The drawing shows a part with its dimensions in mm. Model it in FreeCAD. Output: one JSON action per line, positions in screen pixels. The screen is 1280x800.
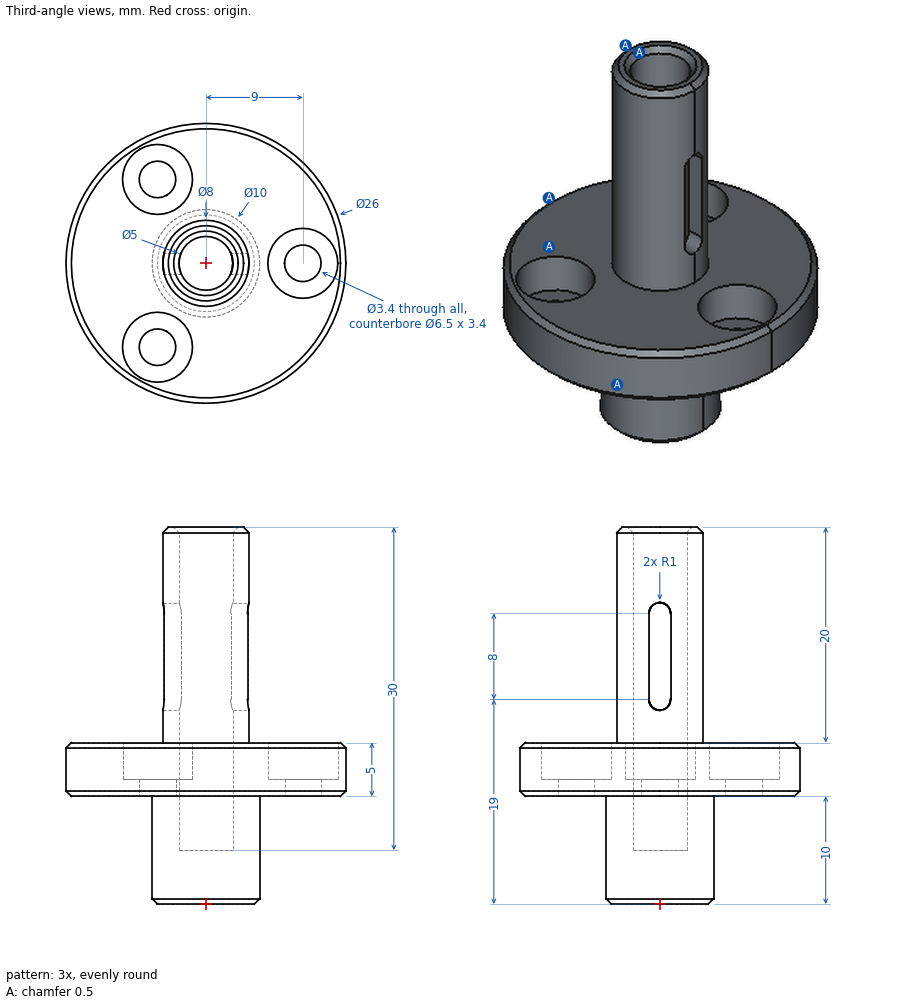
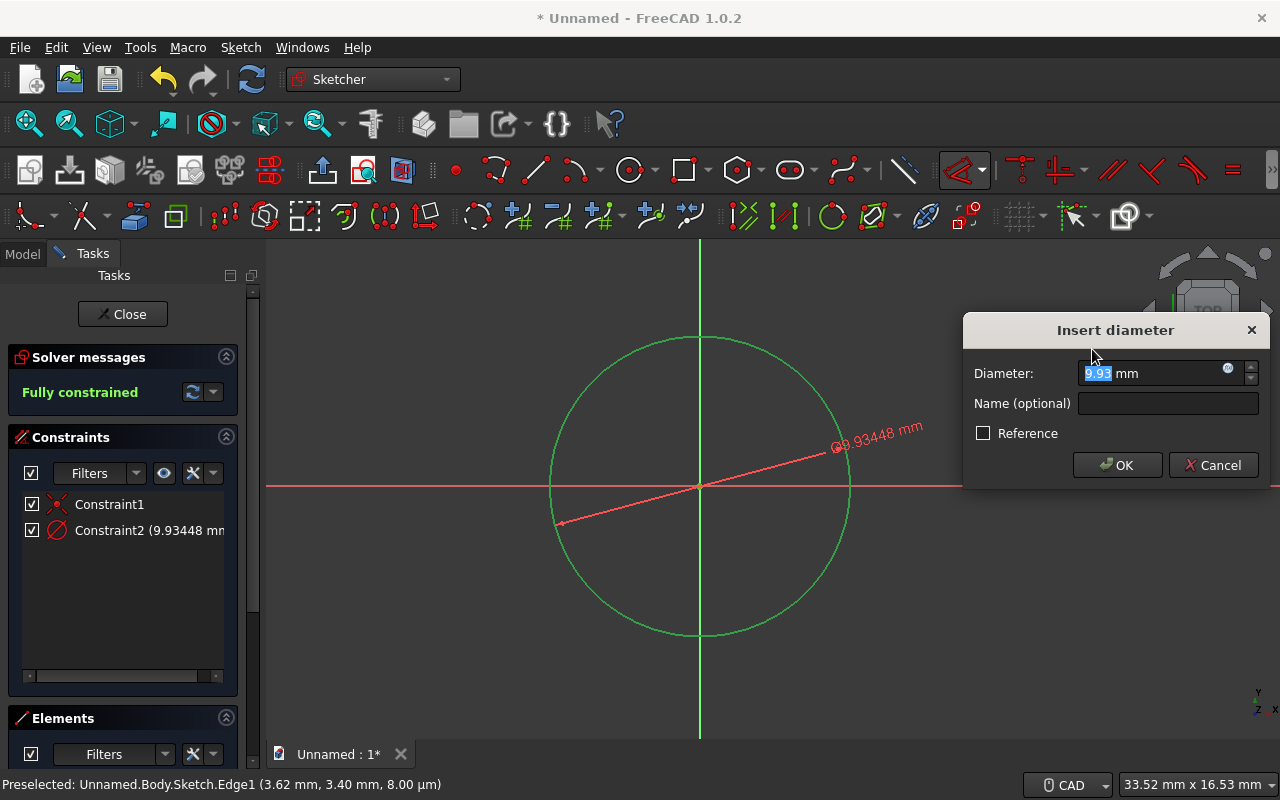
{"action": "type", "text": "10"}
{"action": "key", "text": "Return"}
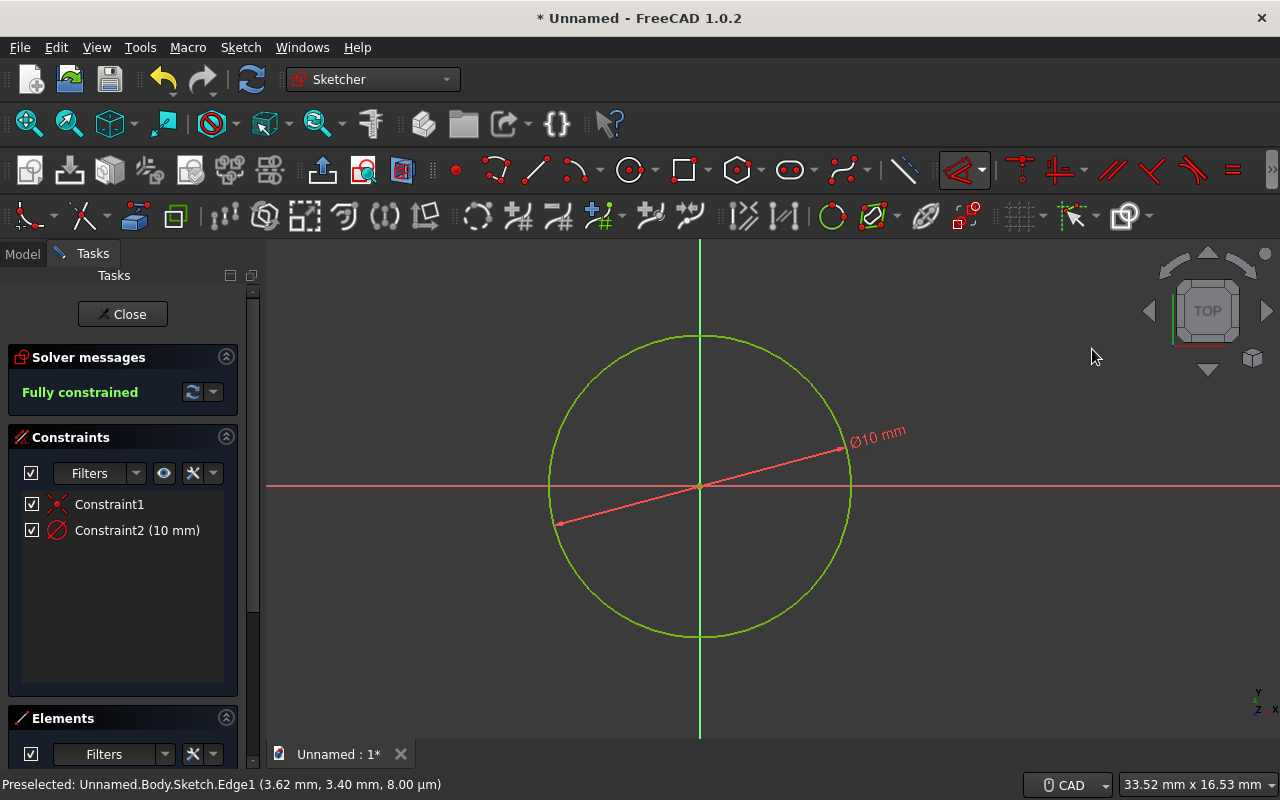
{"action": "left_click", "coordinate": [123, 314]}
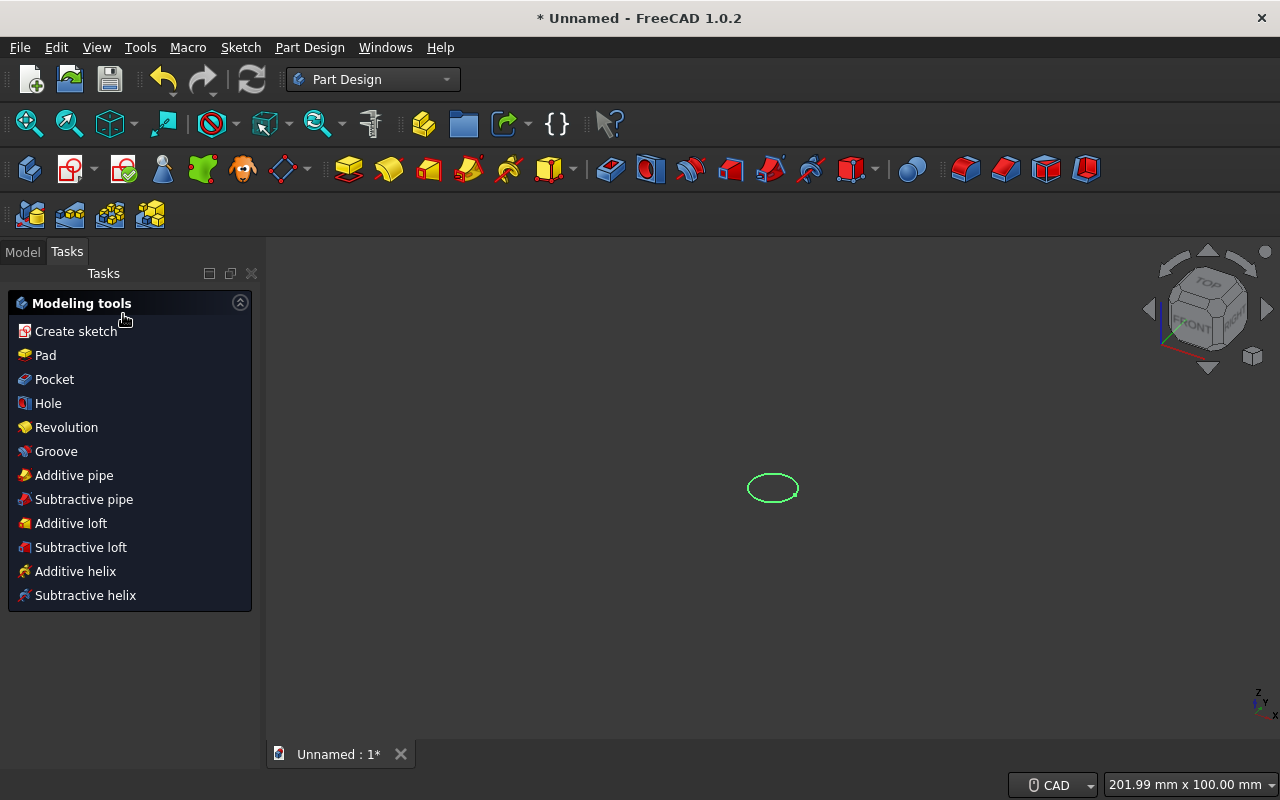
{"action": "left_click", "coordinate": [350, 170]}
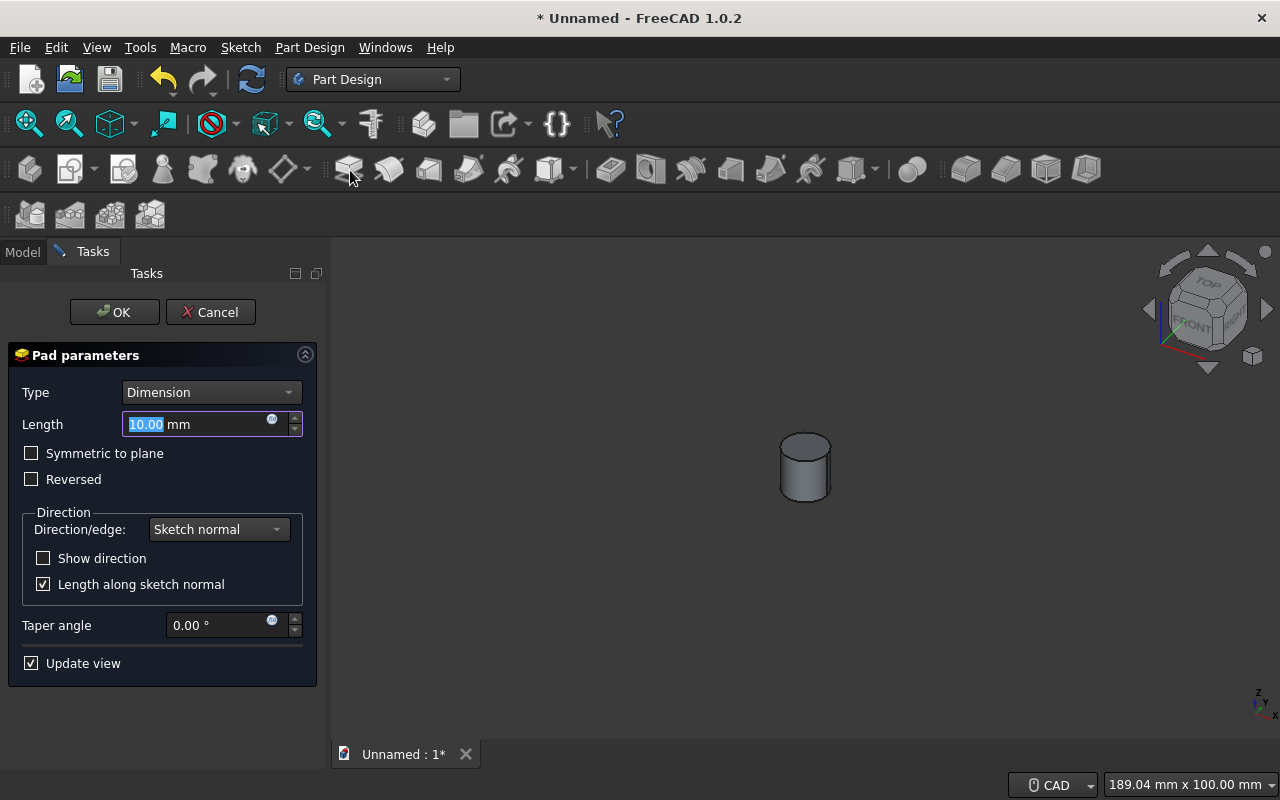
{"action": "type", "text": "10"}
{"action": "key", "text": "Tab"}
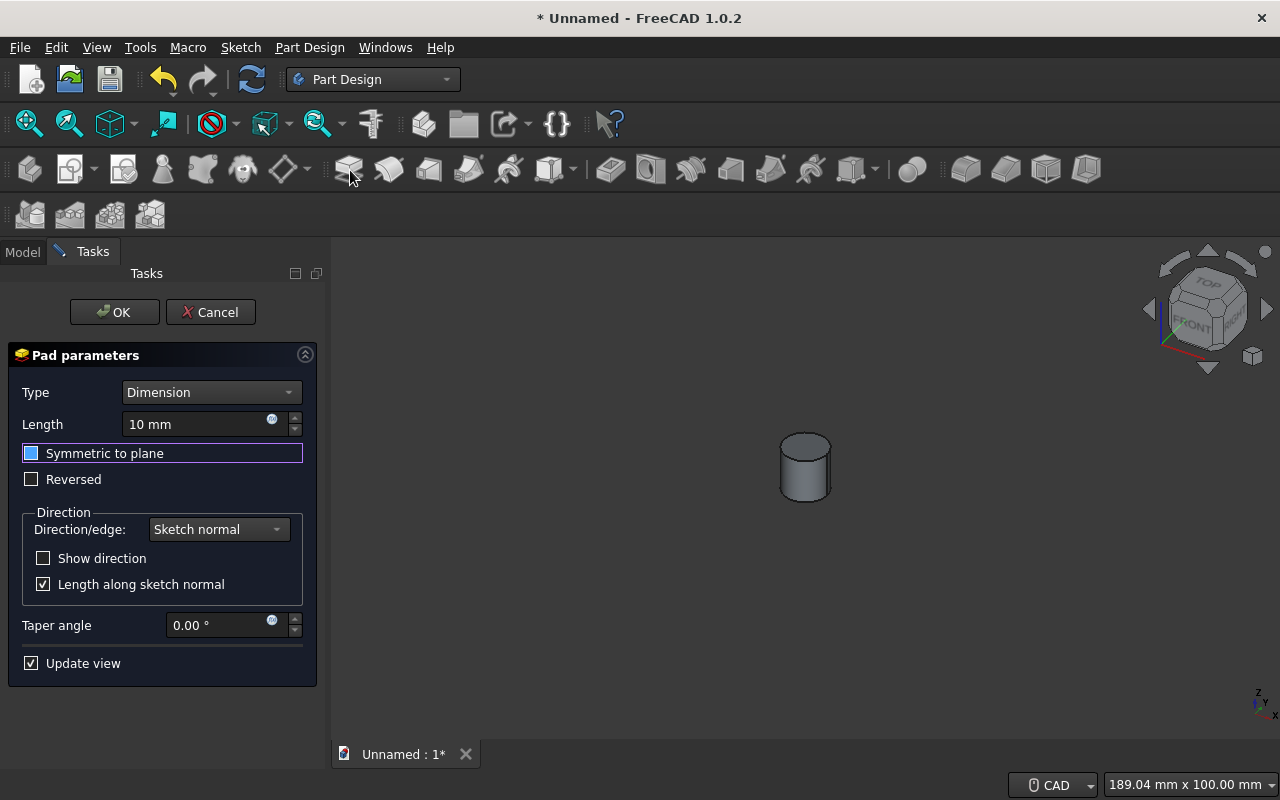
{"action": "left_click", "coordinate": [115, 312]}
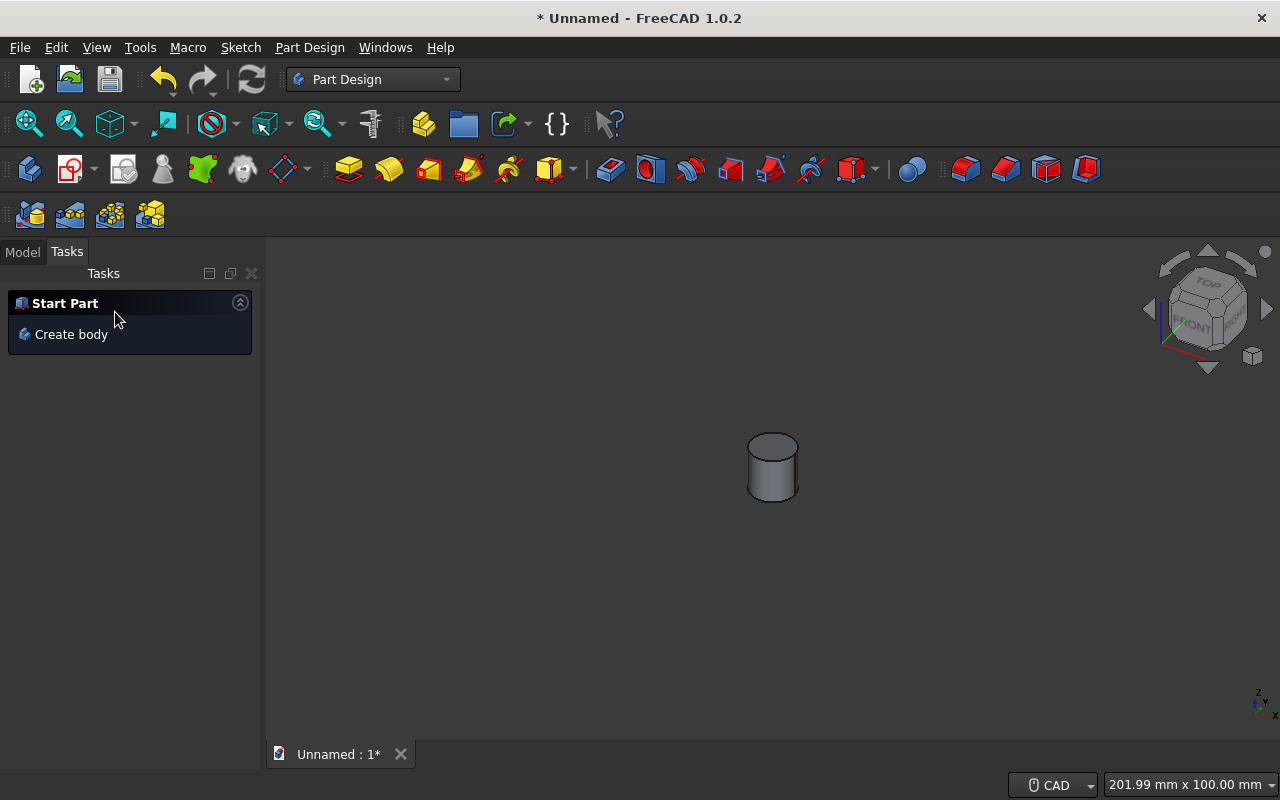
{"action": "left_click", "coordinate": [30, 124]}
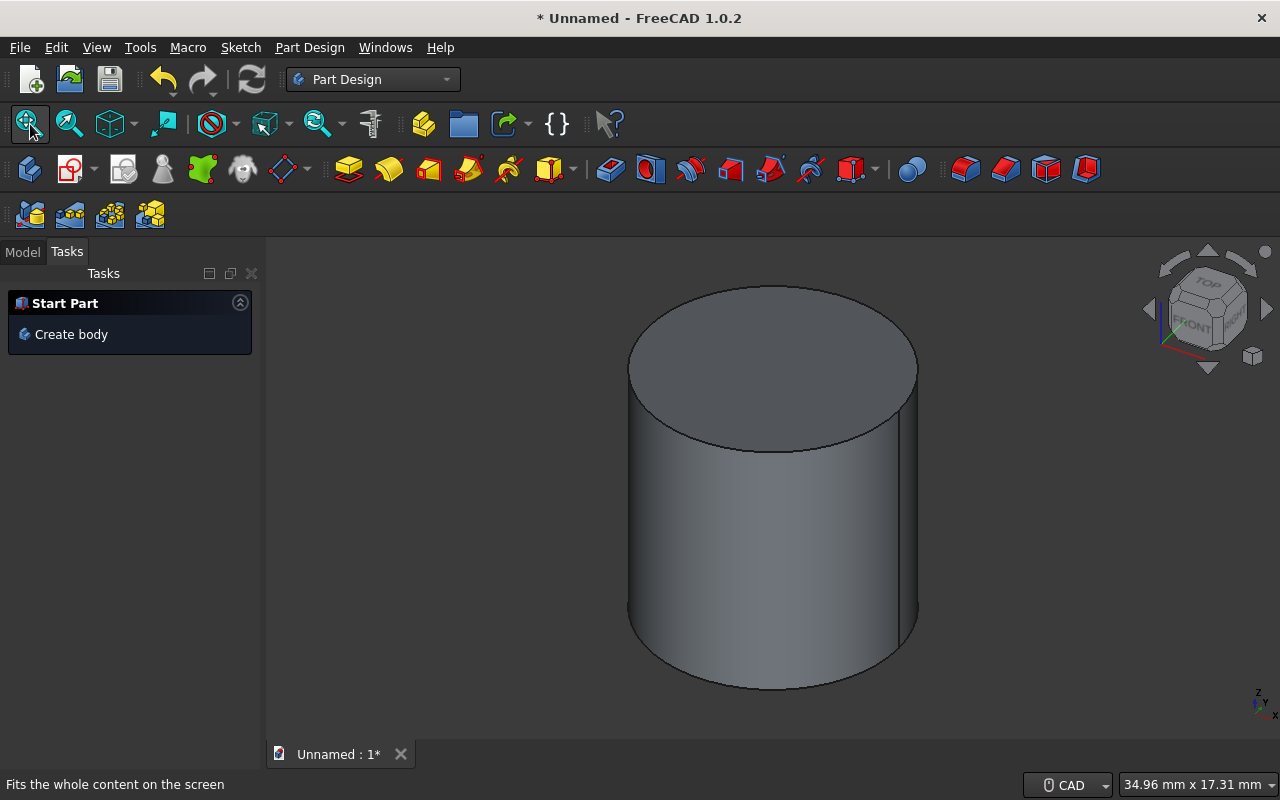
{"action": "left_click", "coordinate": [773, 368]}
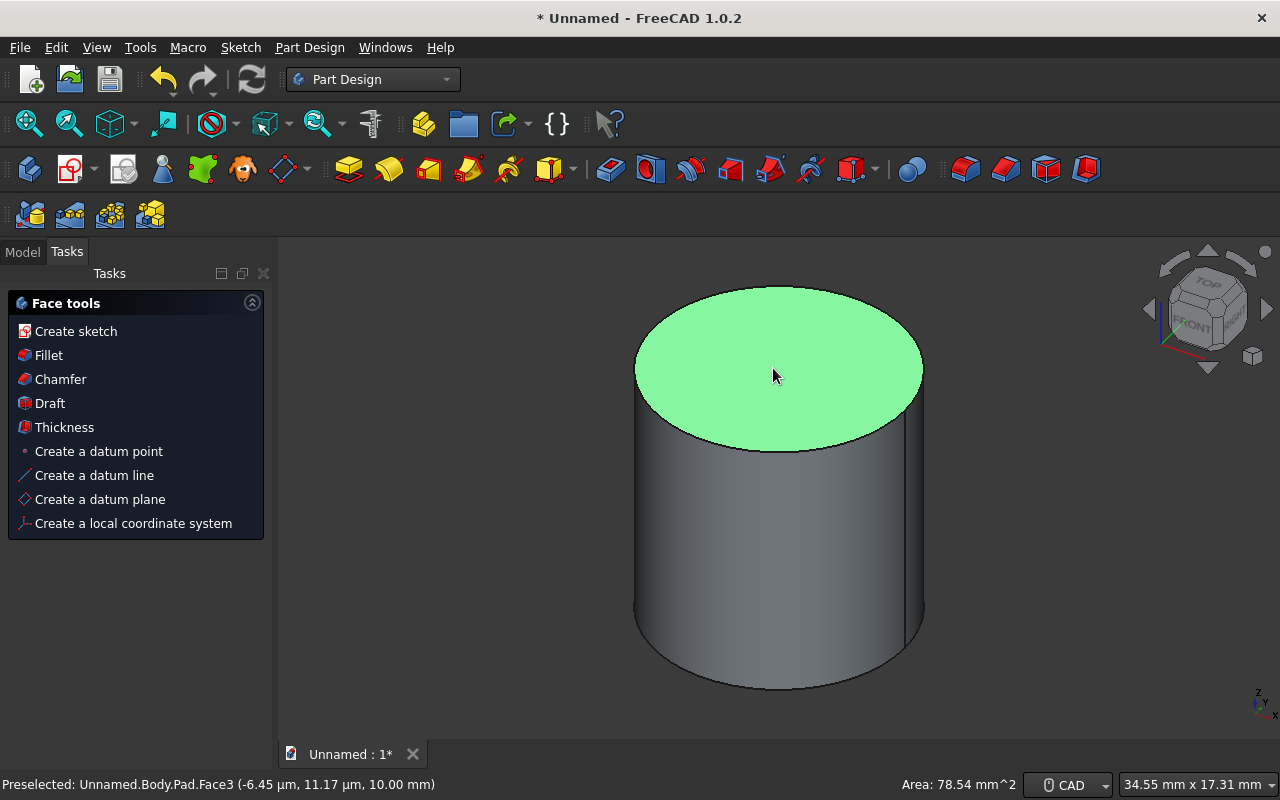
{"action": "left_click", "coordinate": [70, 170]}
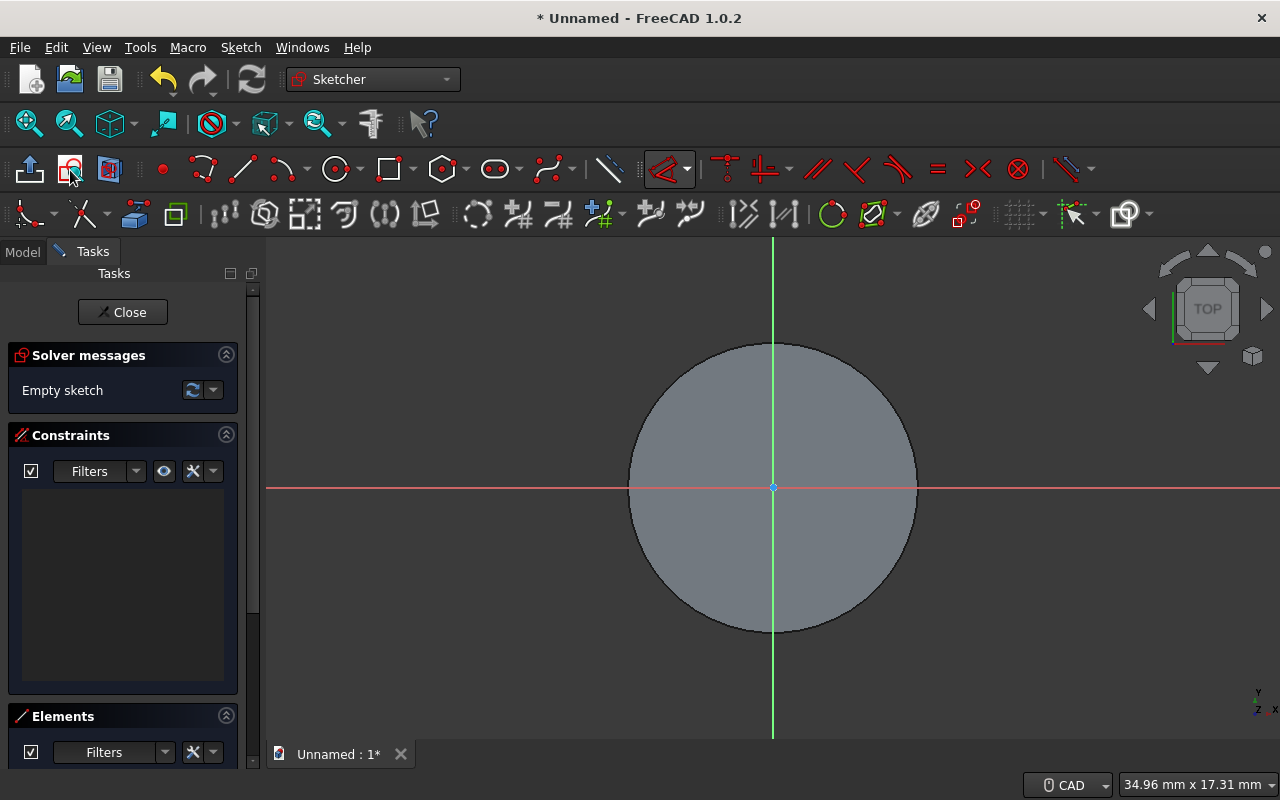
{"action": "scroll", "coordinate": [649, 488], "scroll_direction": "down", "scroll_amount": 4}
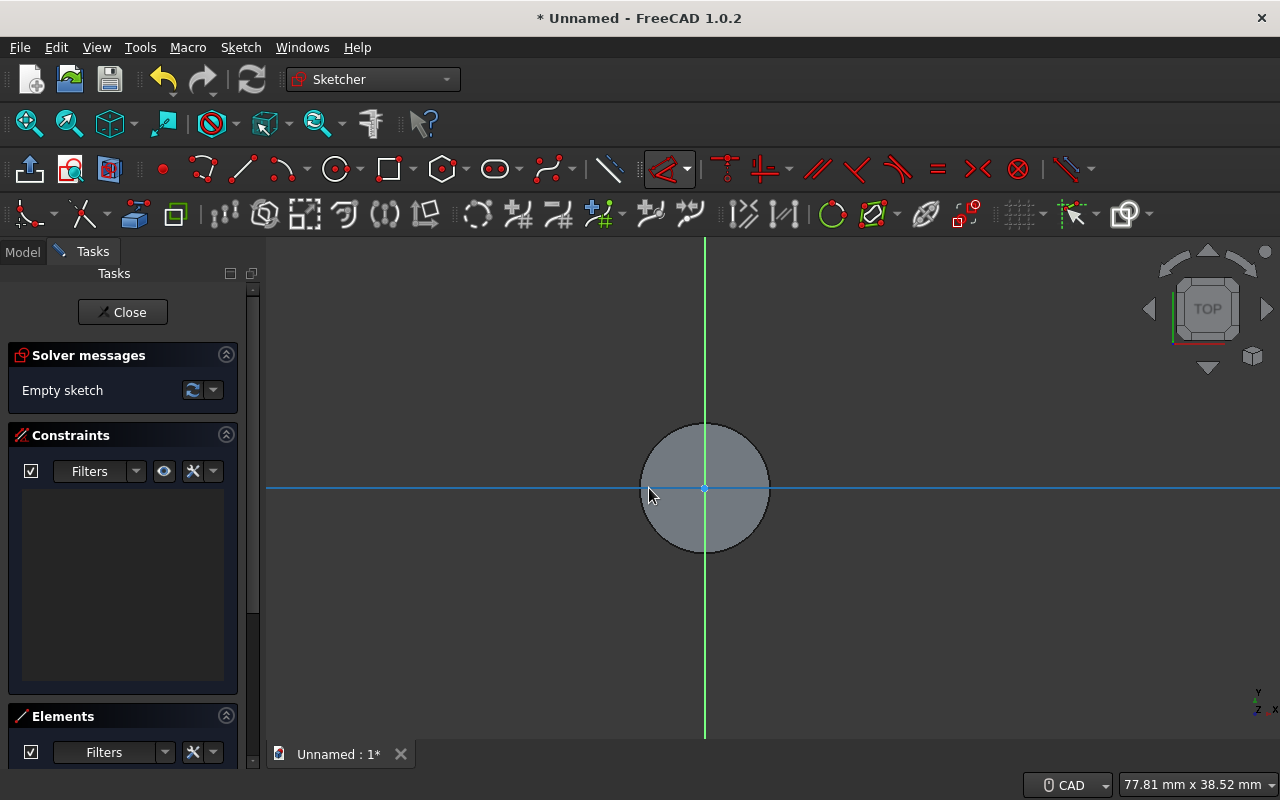
{"action": "left_click", "coordinate": [336, 170]}